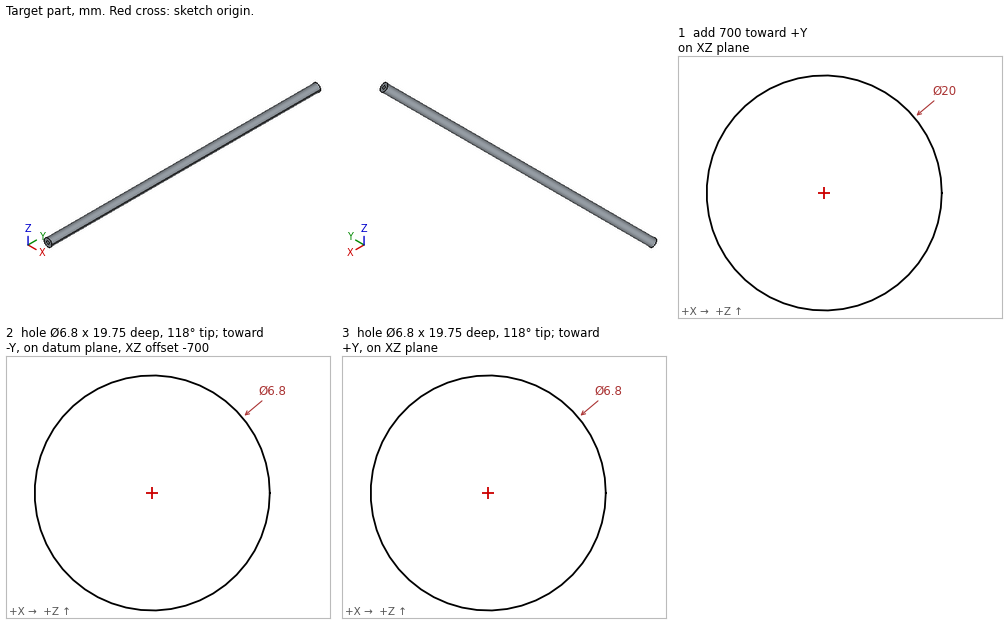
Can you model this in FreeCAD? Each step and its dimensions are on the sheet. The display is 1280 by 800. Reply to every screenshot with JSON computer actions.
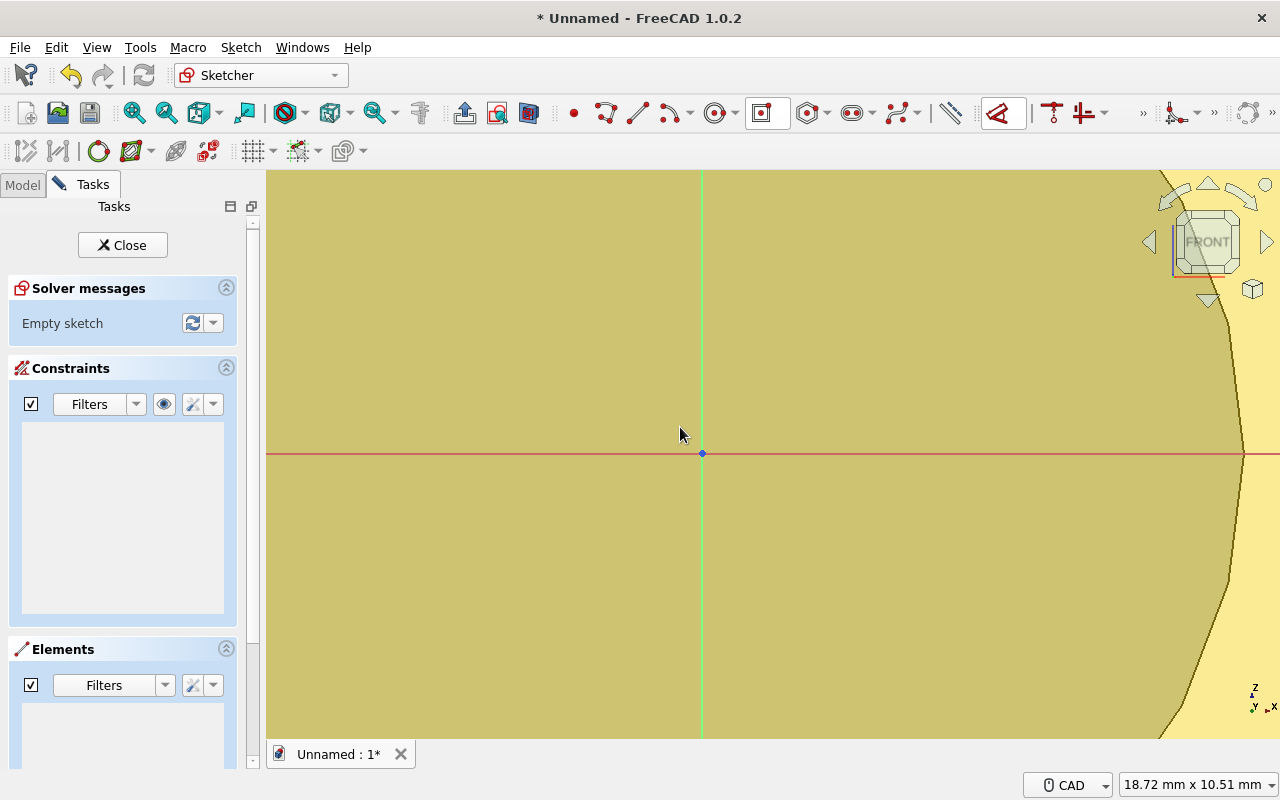
{"action": "left_click", "coordinate": [716, 114]}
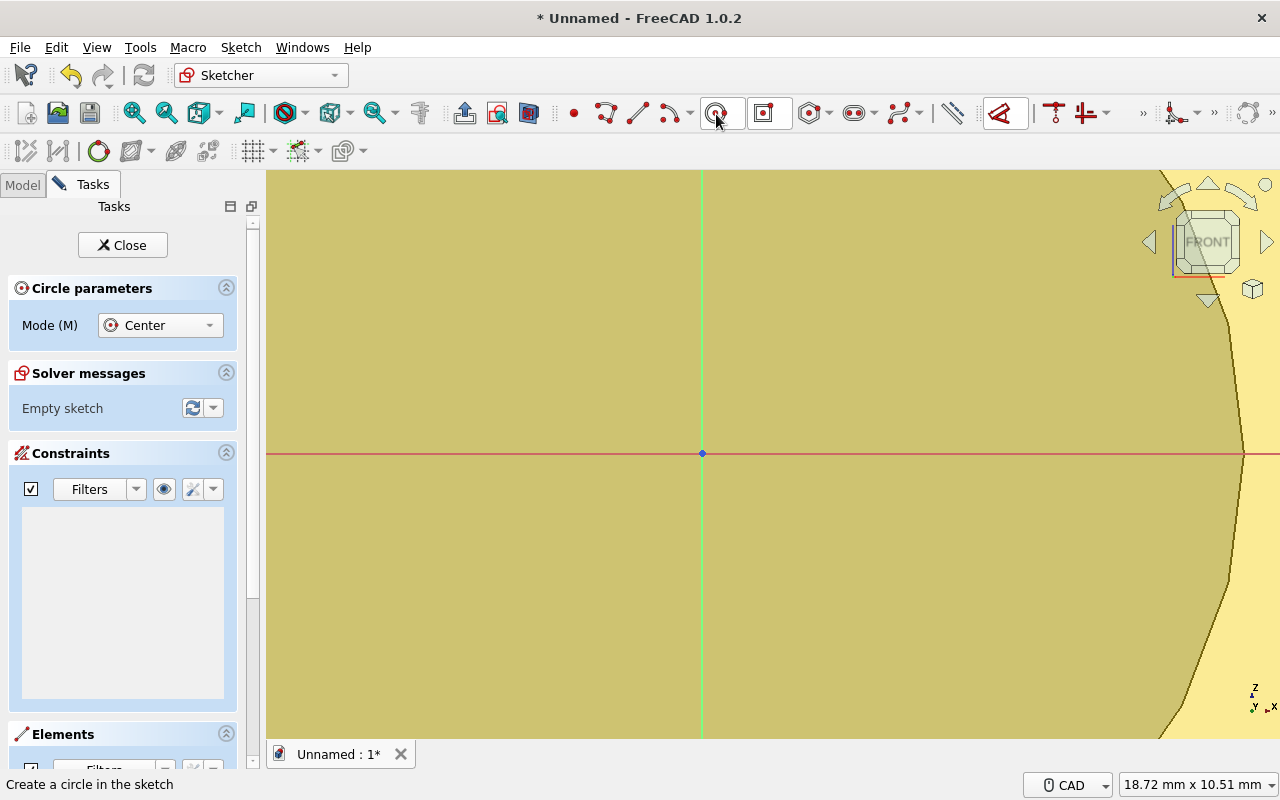
{"action": "left_click", "coordinate": [702, 454]}
{"action": "mouse_move", "coordinate": [833, 324]}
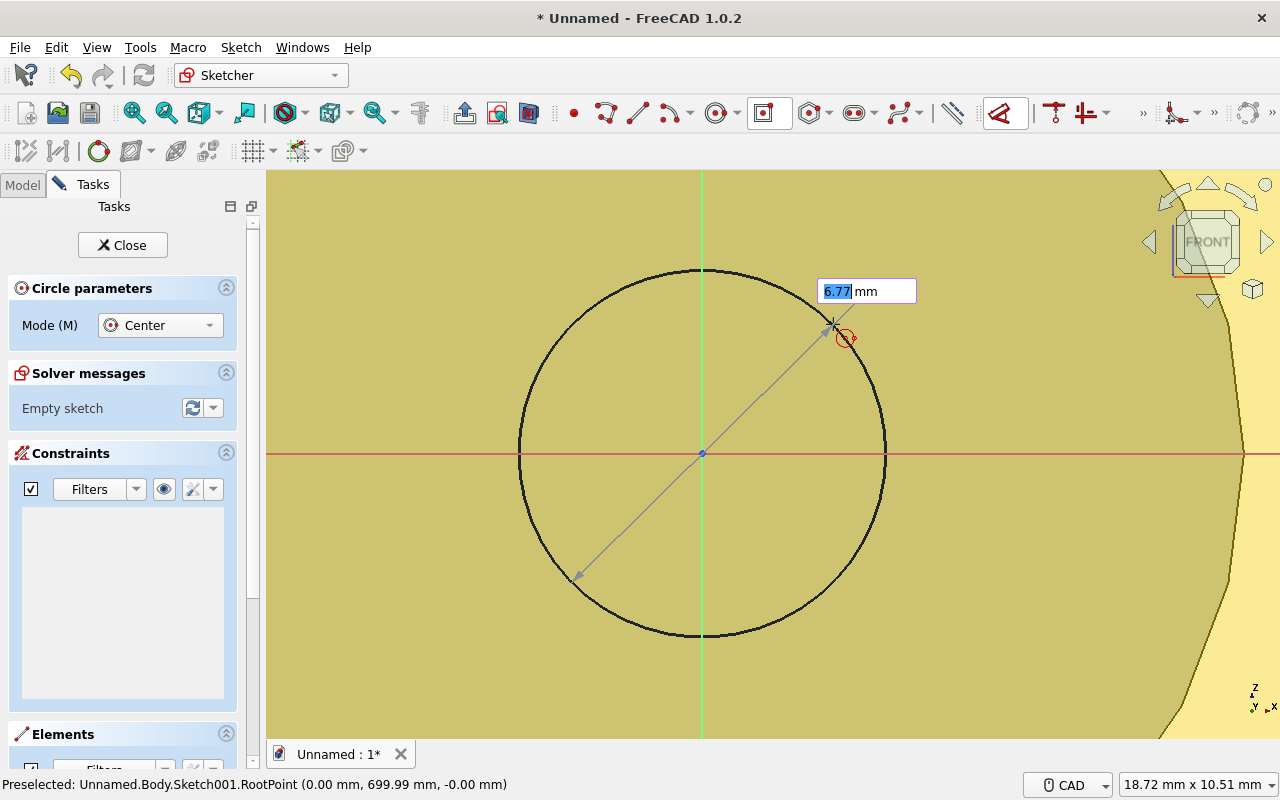
{"action": "type", "text": "6.8"}
{"action": "key", "text": "Return"}
{"action": "key", "text": "Escape"}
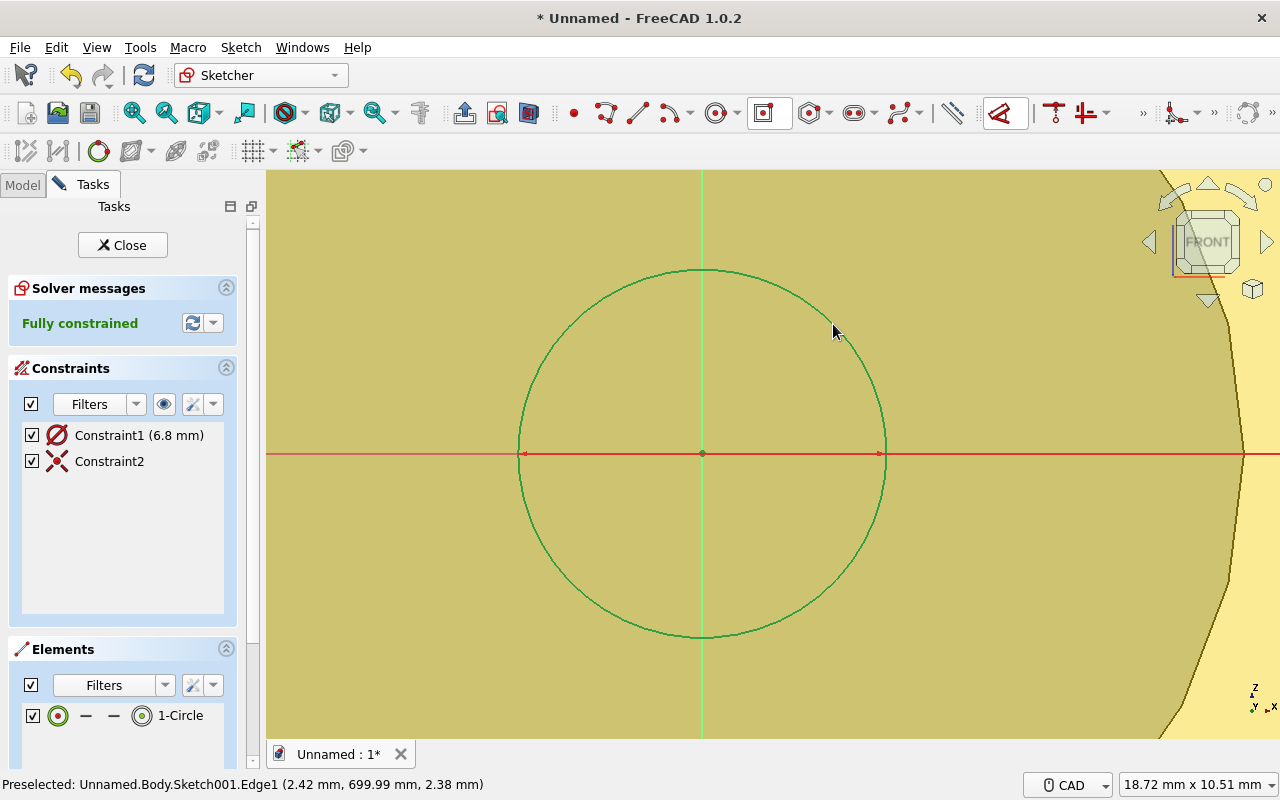
{"action": "left_click", "coordinate": [123, 245]}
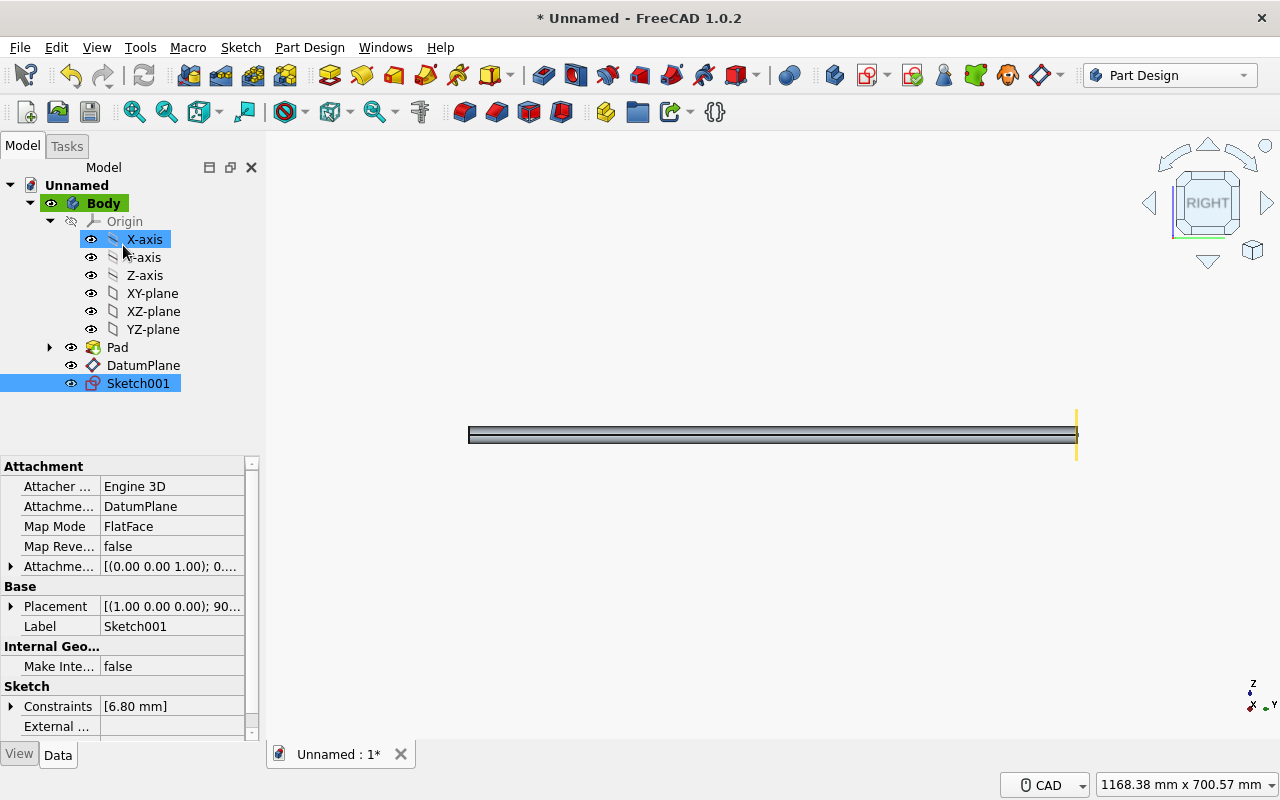
{"action": "left_click", "coordinate": [576, 76]}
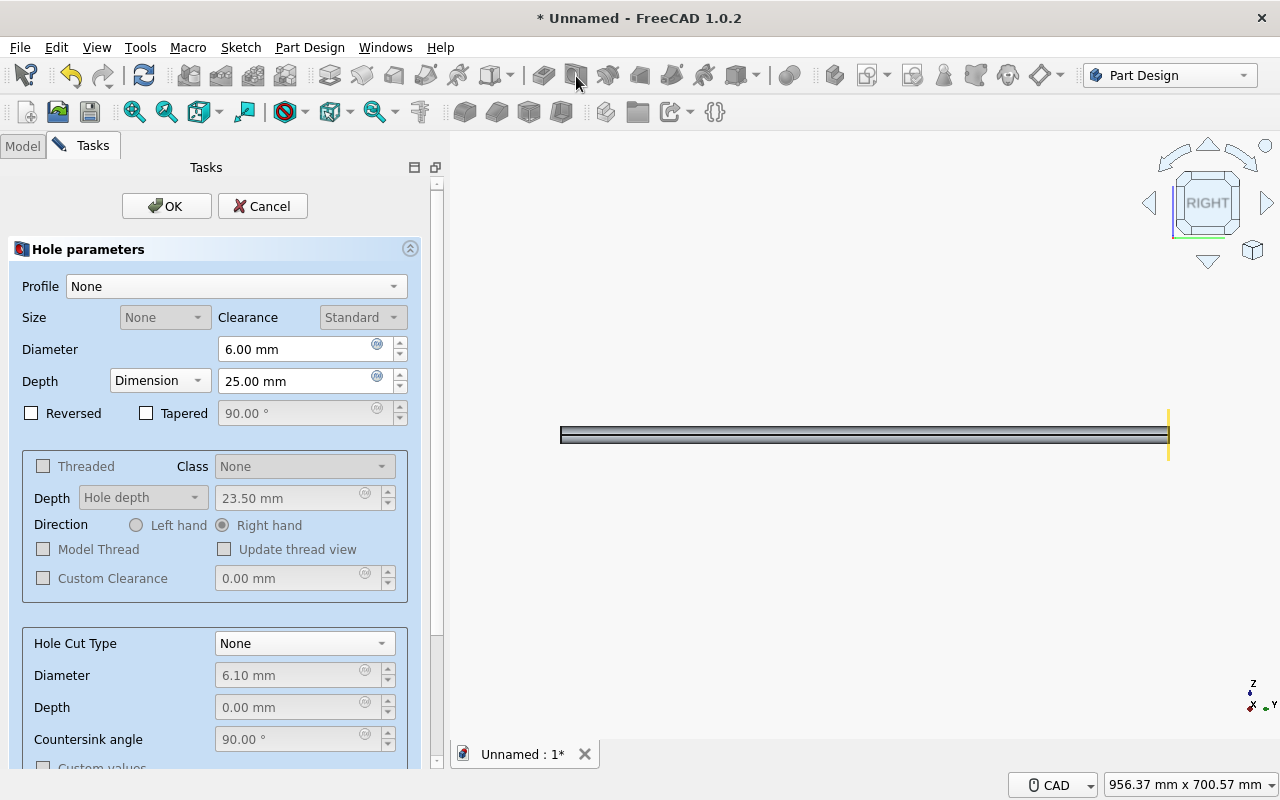
{"action": "triple_click", "coordinate": [305, 349]}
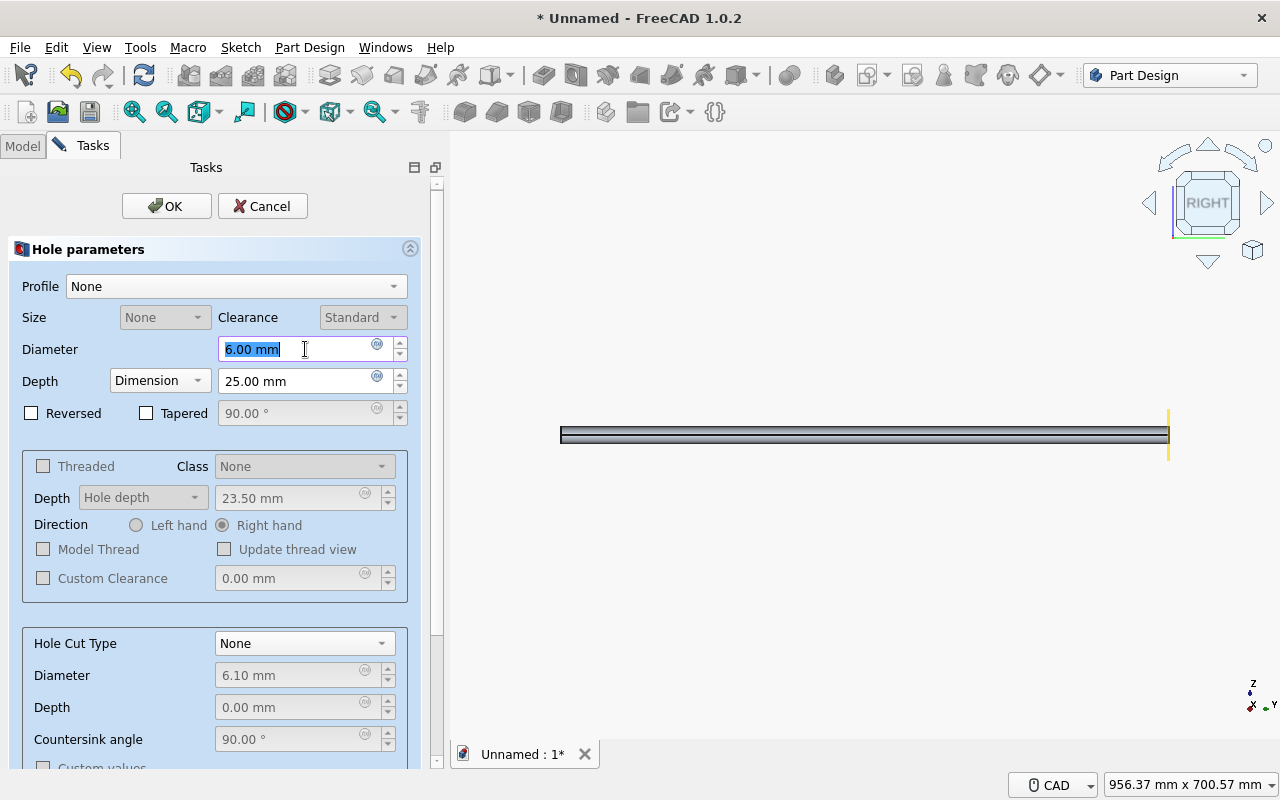
{"action": "type", "text": "6.8"}
{"action": "key", "text": "Tab"}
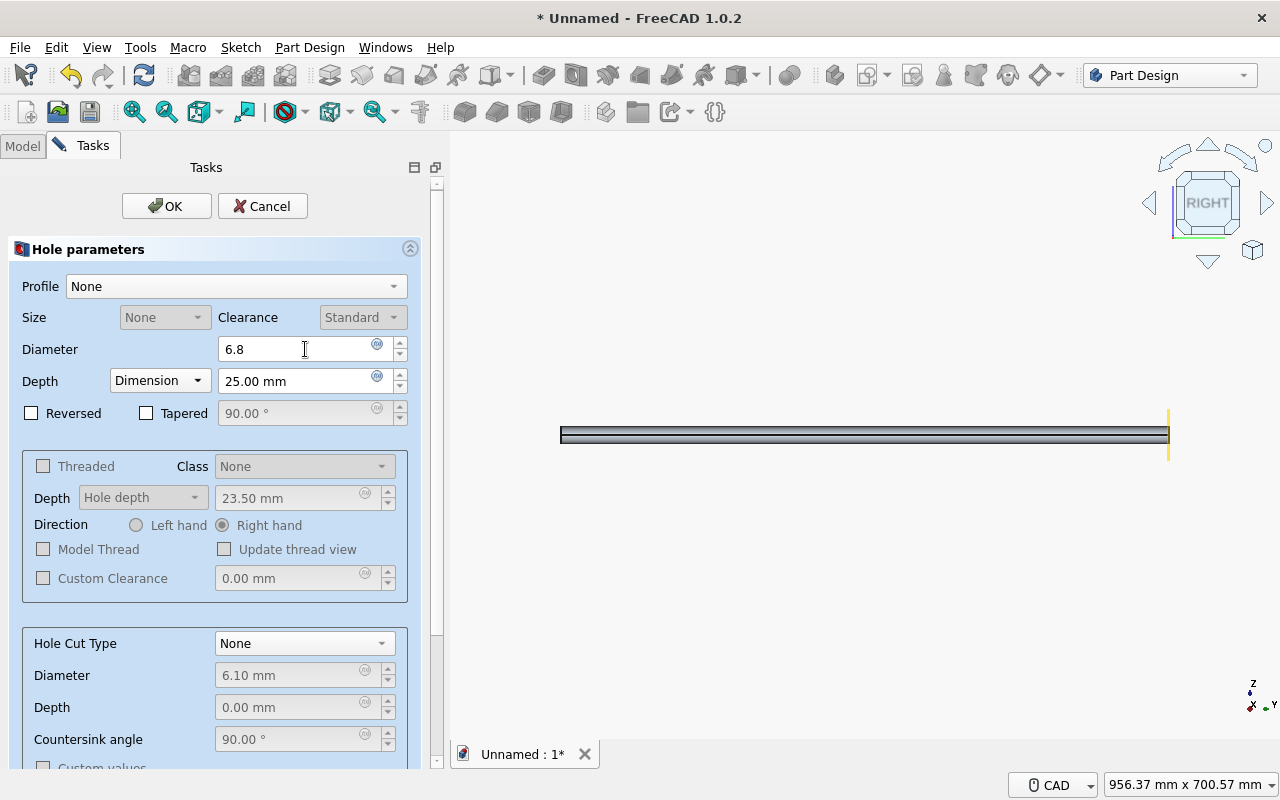
{"action": "triple_click", "coordinate": [305, 381]}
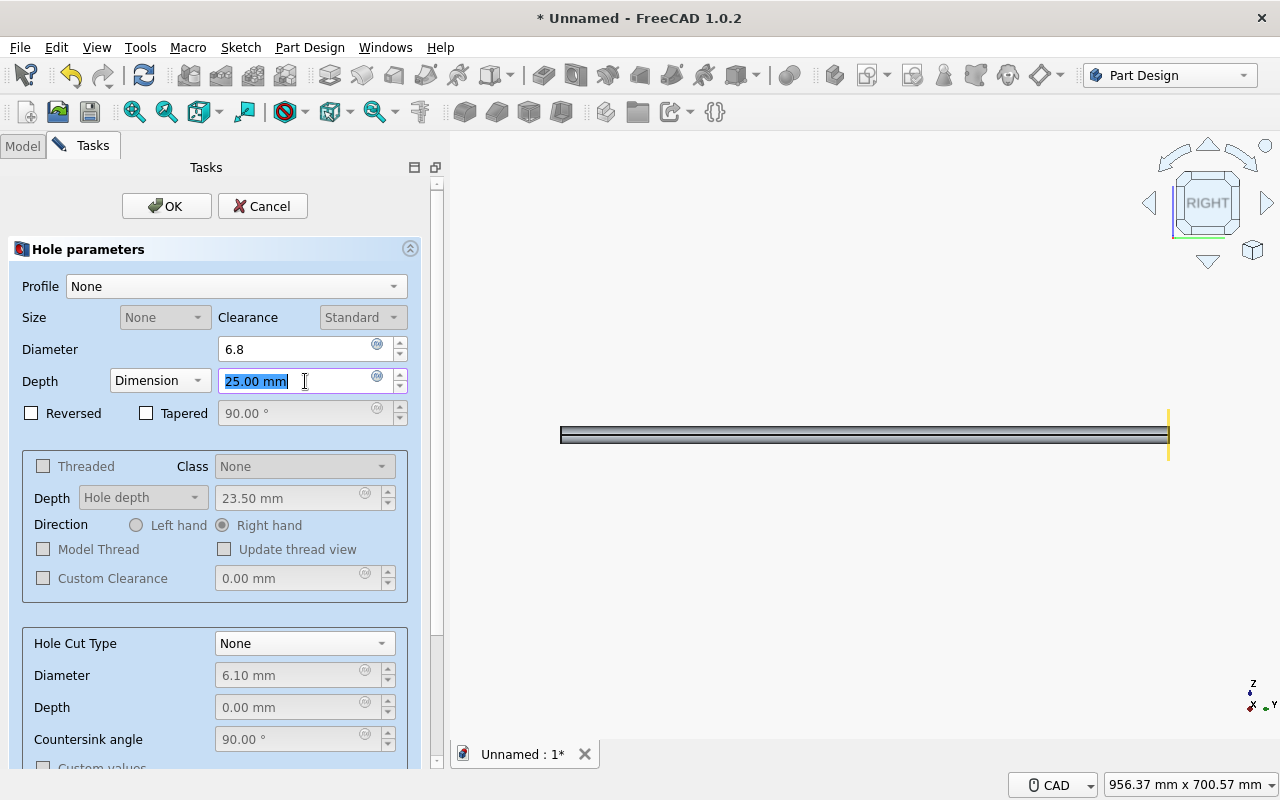
{"action": "type", "text": "19.75"}
{"action": "key", "text": "Tab"}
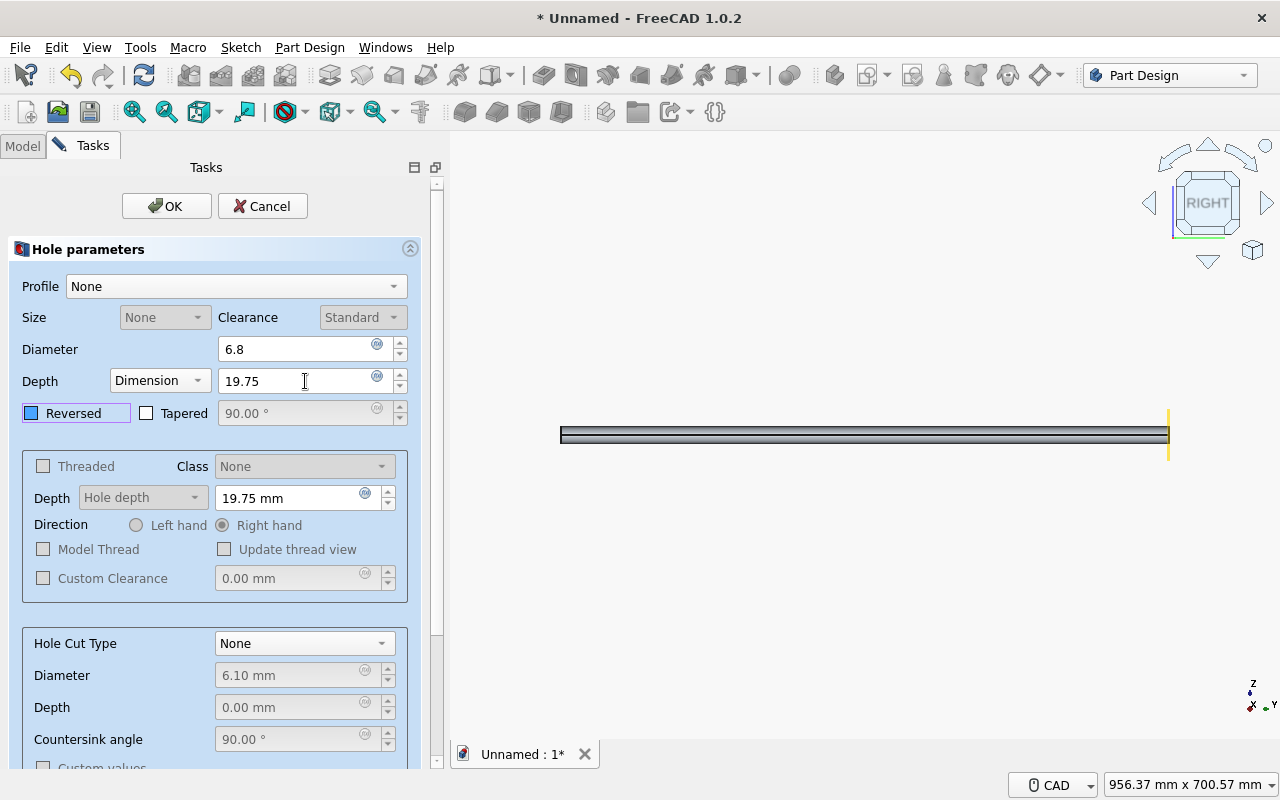
{"action": "left_click", "coordinate": [30, 413]}